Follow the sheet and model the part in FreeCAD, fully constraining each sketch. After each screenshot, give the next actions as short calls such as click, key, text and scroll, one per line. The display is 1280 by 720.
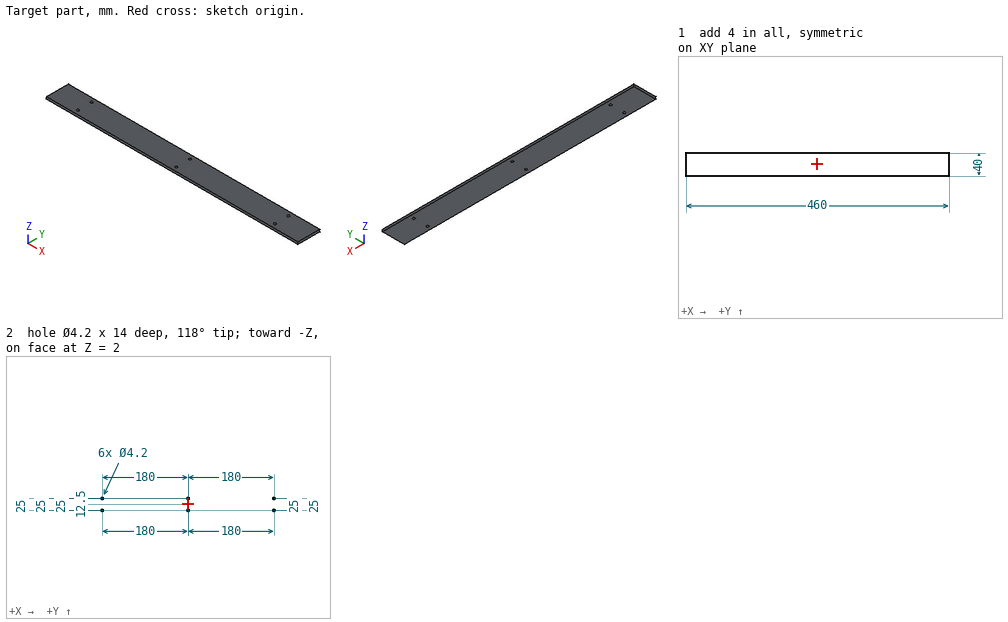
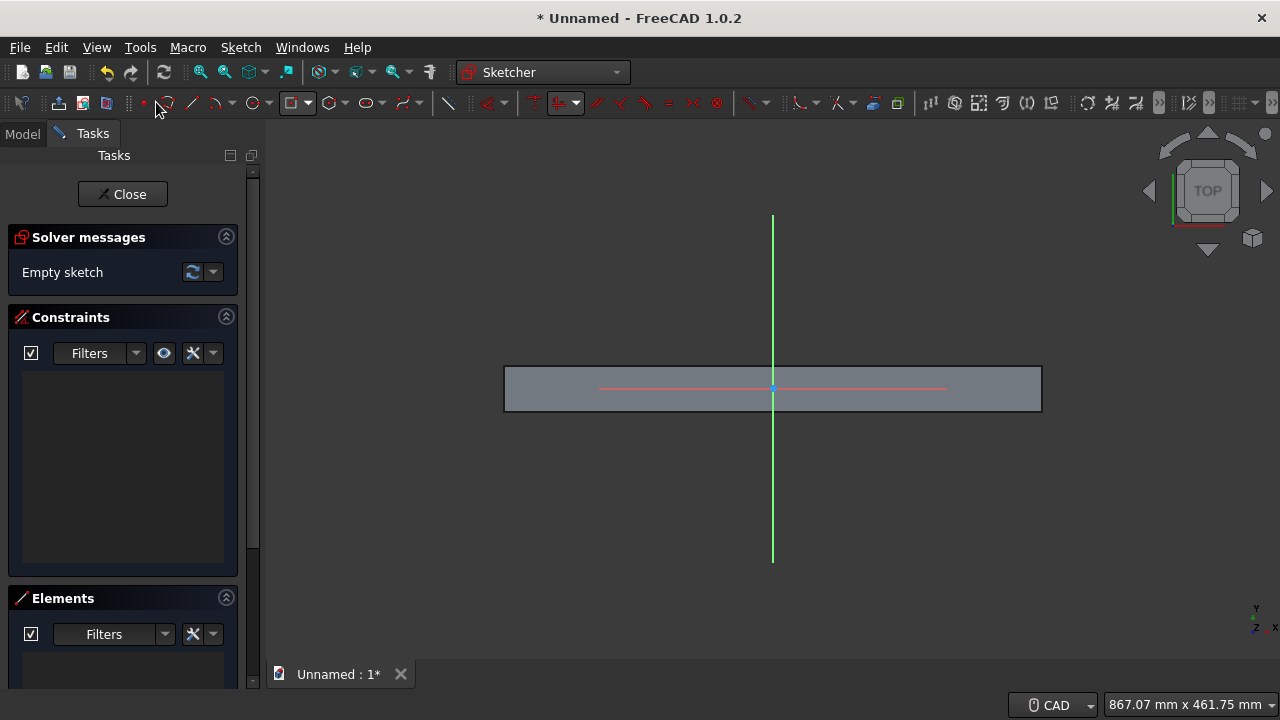
scroll(912, 389, up, 2)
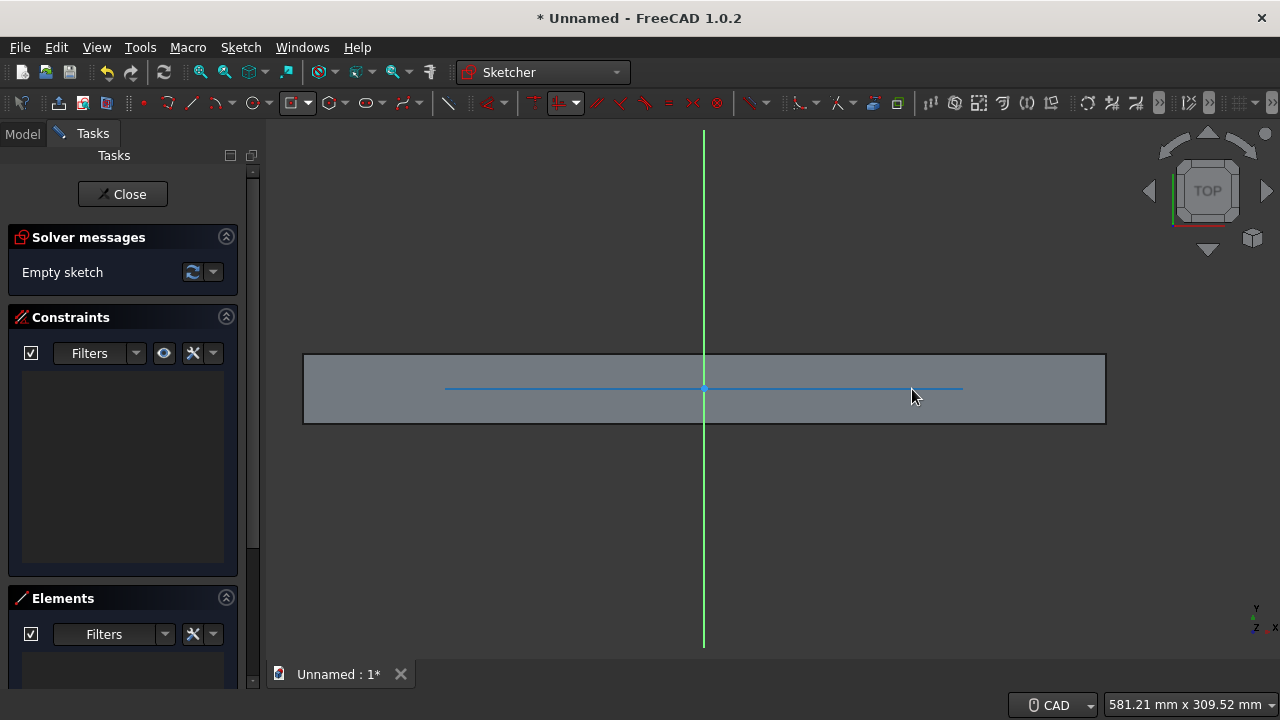
key(g)
key(c)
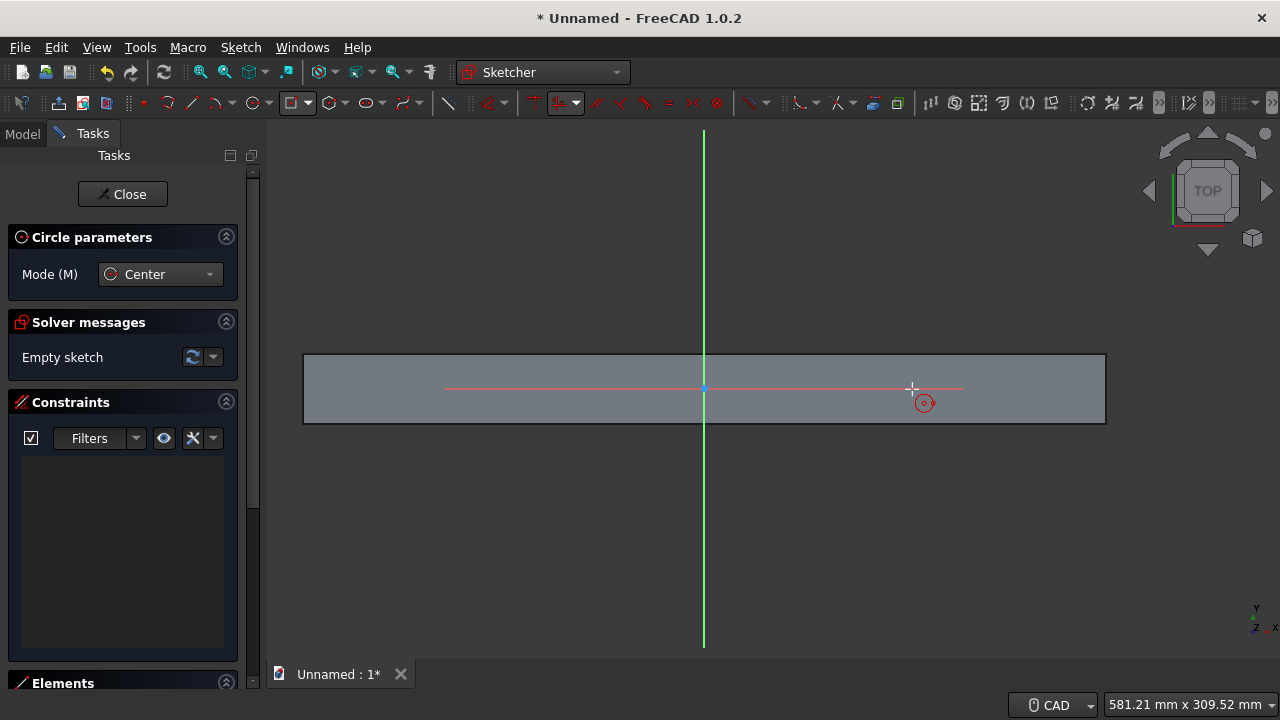
scroll(390, 367, up, 10)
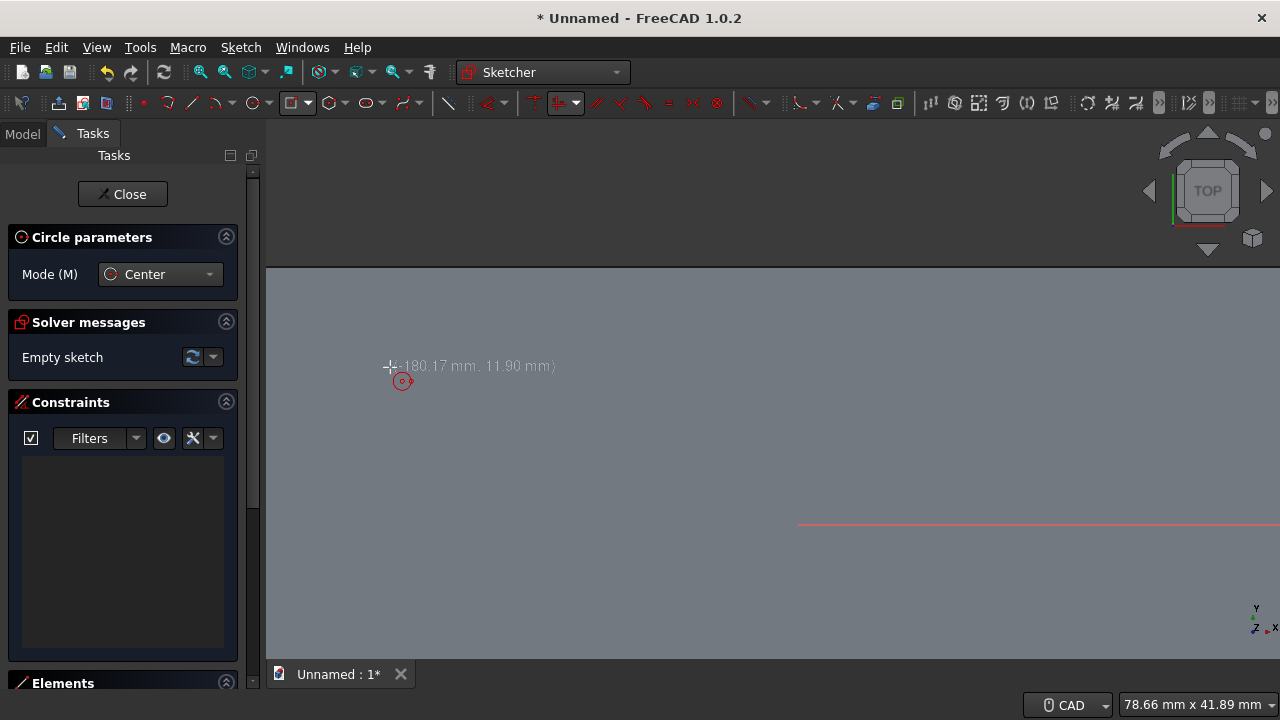
scroll(390, 368, down, 10)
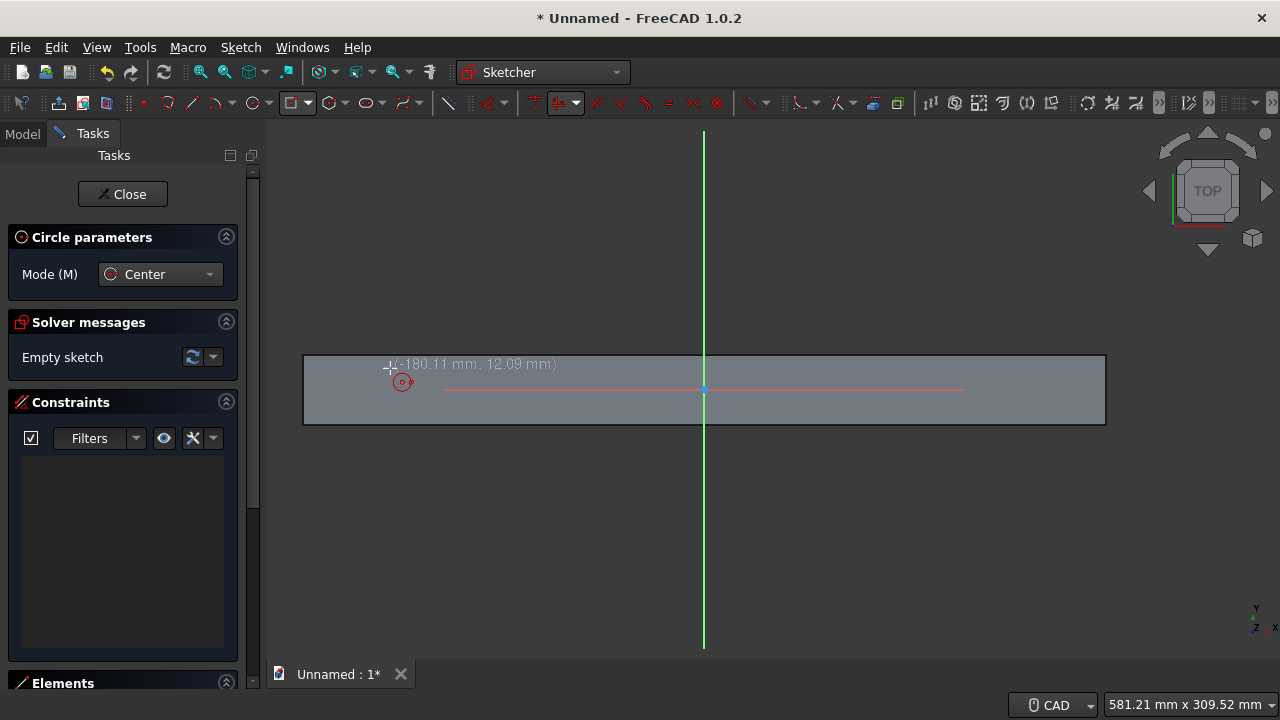
click(390, 368)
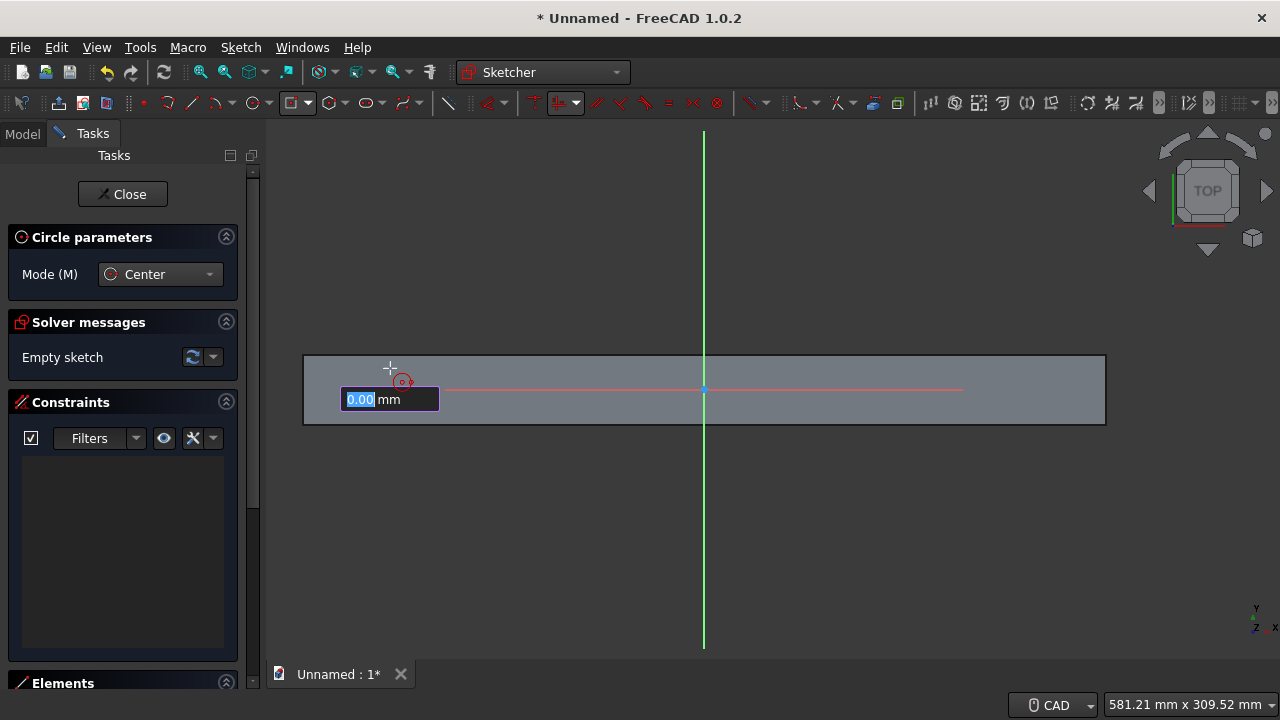
scroll(393, 365, up, 8)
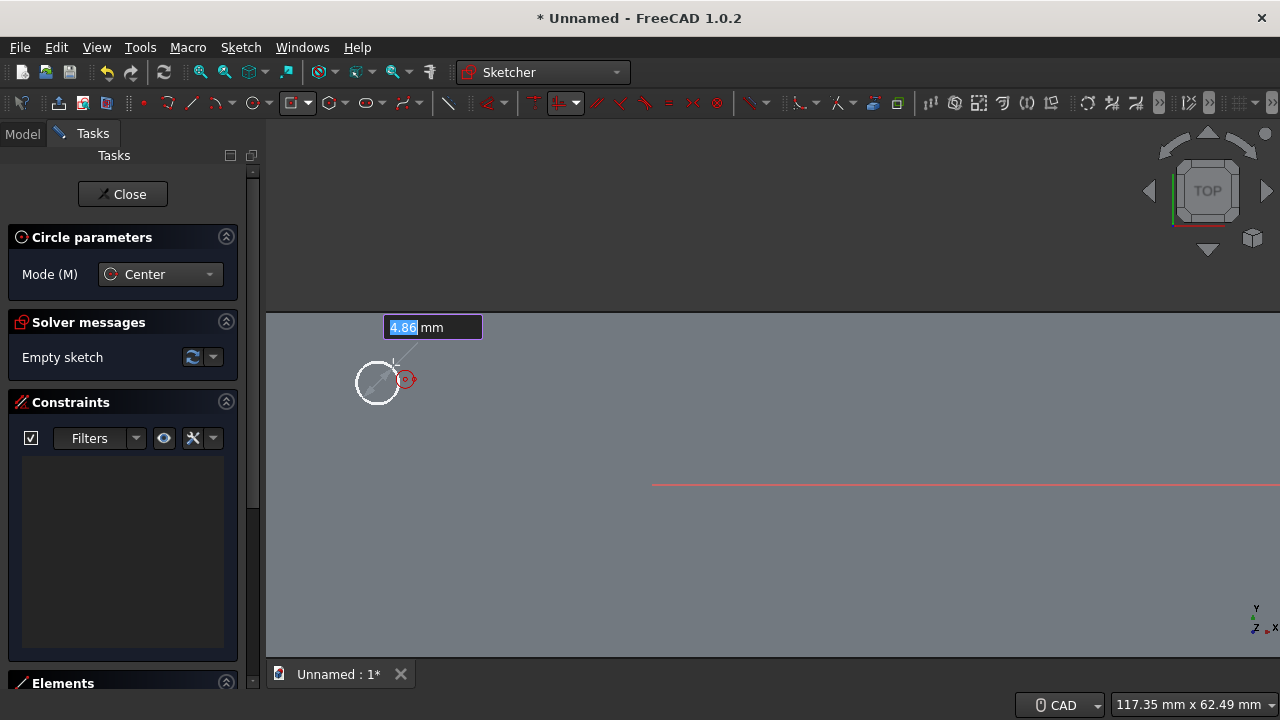
click(392, 364)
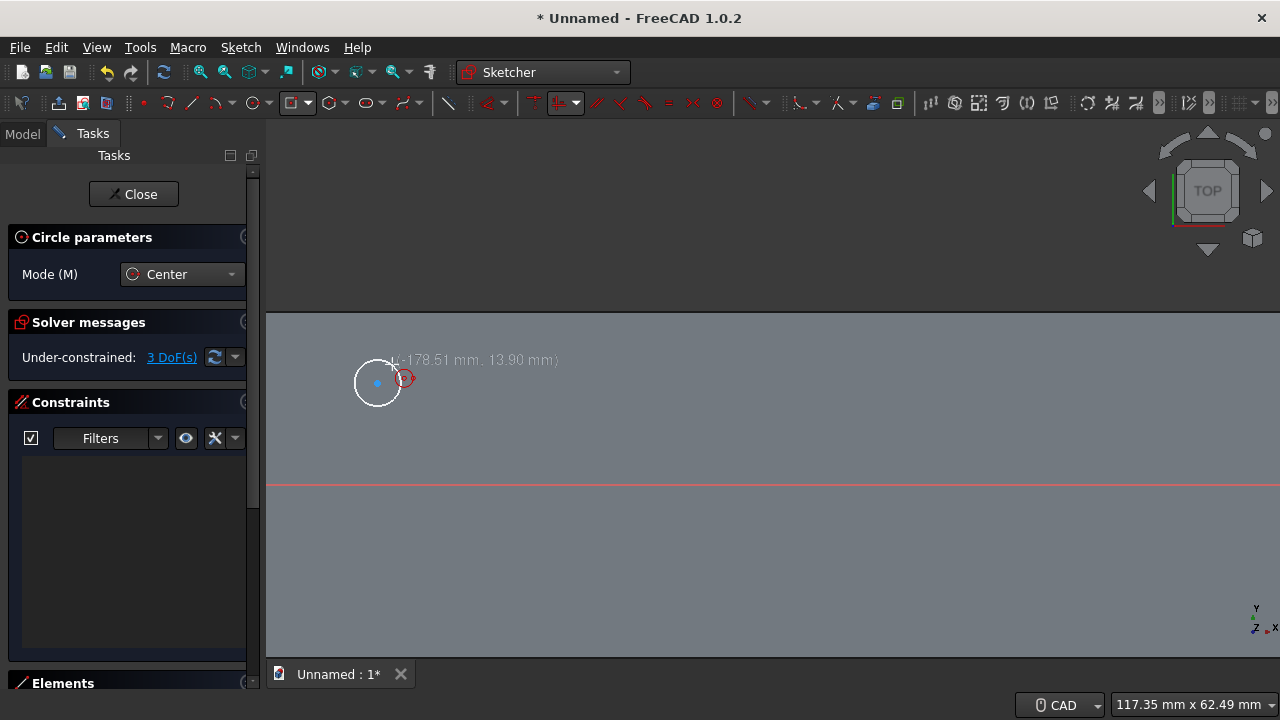
scroll(379, 593, up, 2)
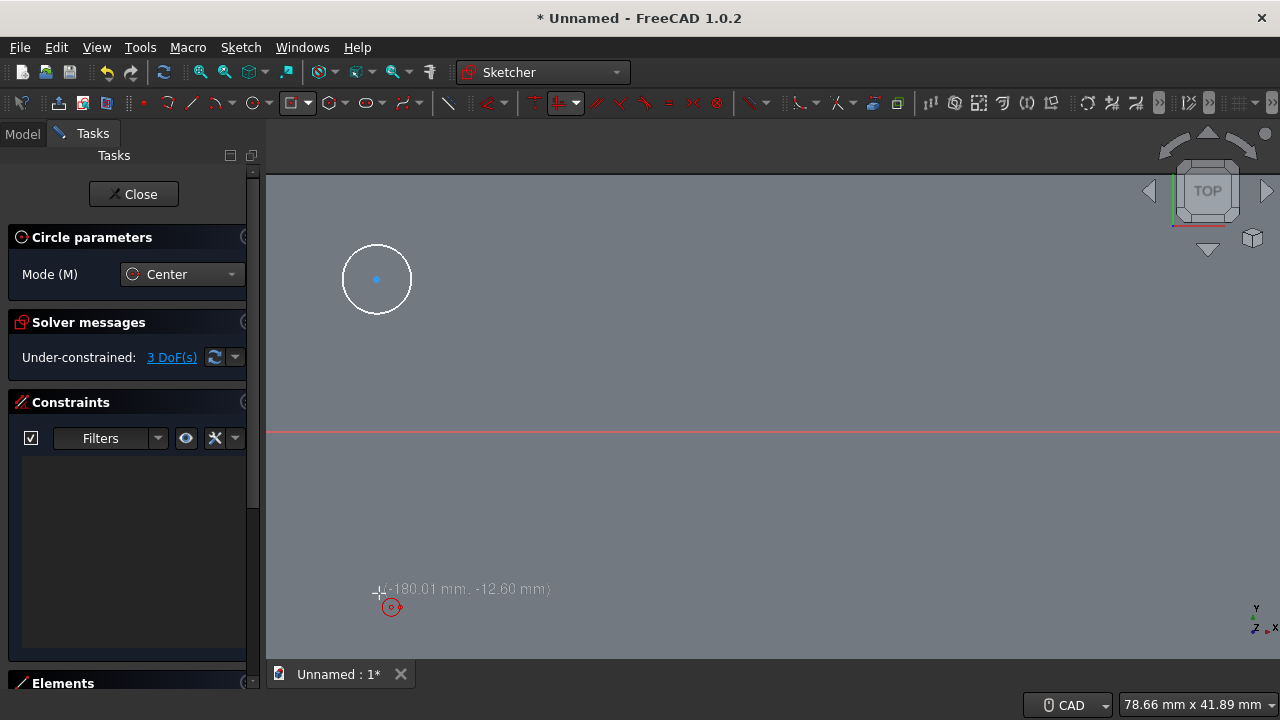
scroll(392, 382, down, 10)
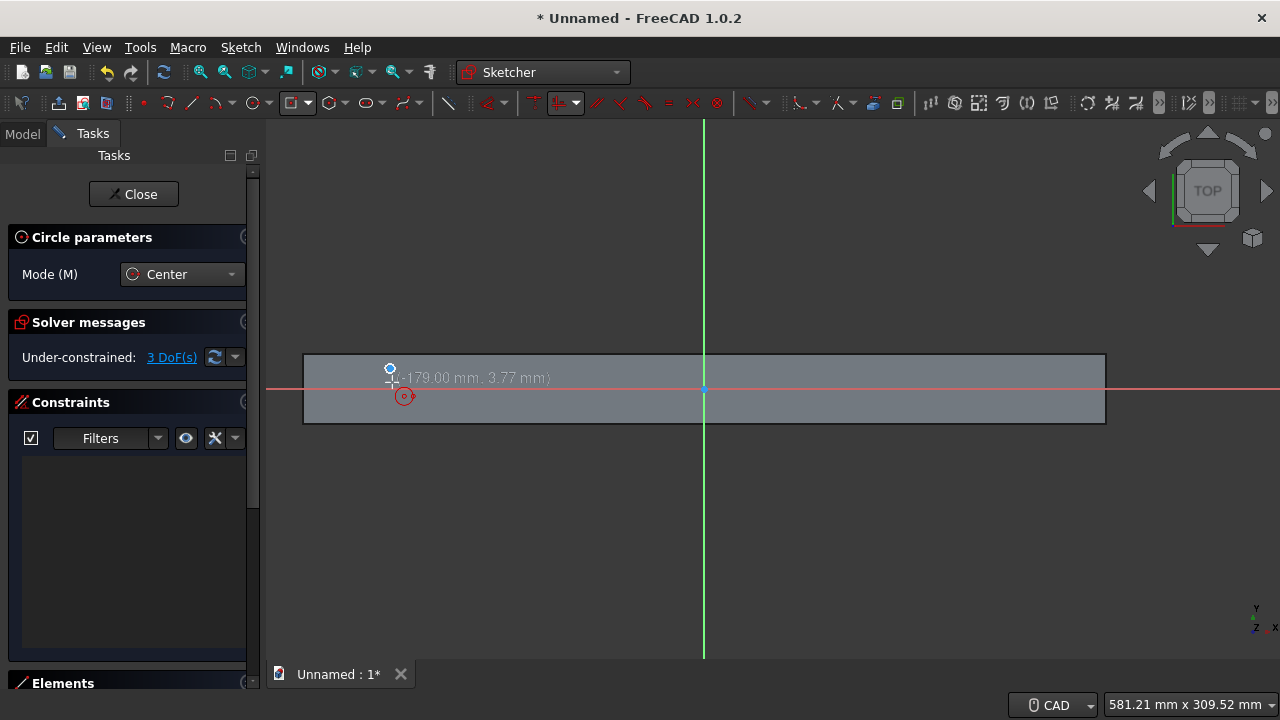
click(390, 411)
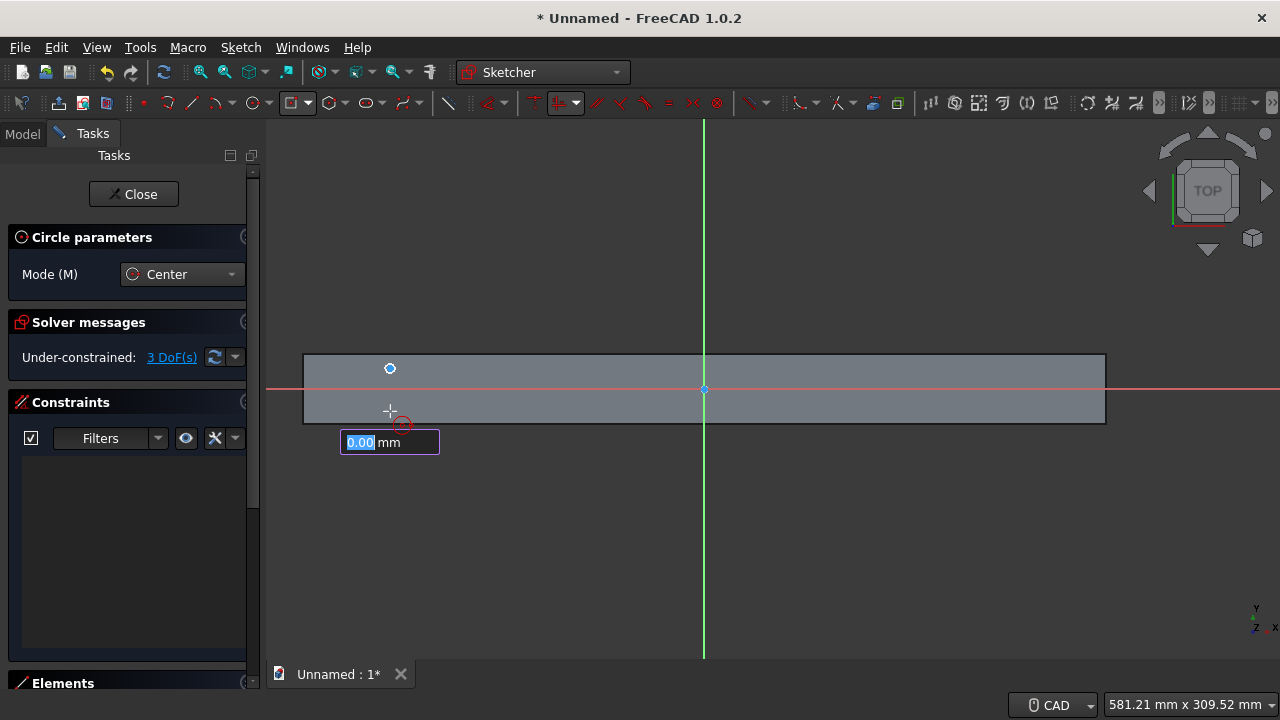
scroll(393, 408, up, 8)